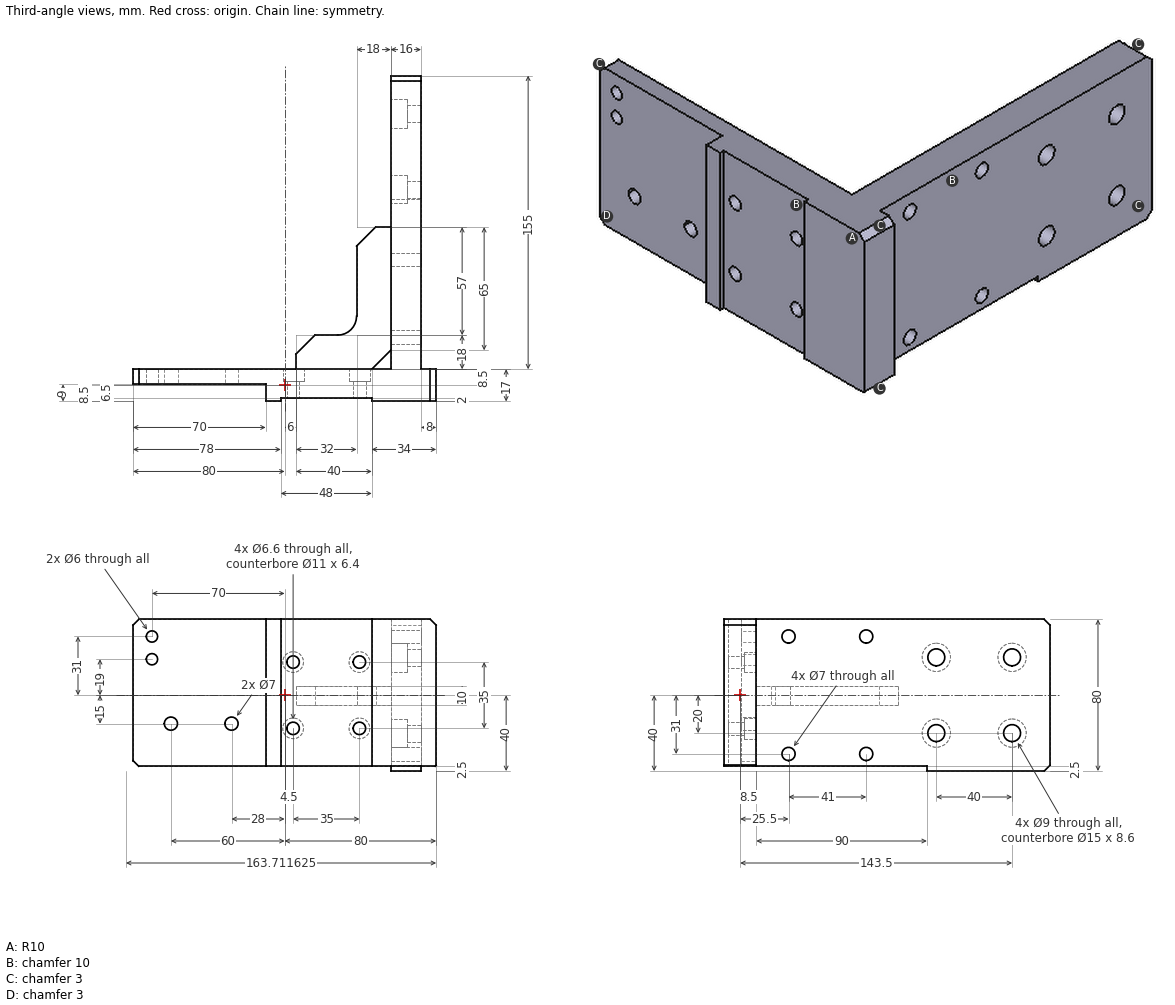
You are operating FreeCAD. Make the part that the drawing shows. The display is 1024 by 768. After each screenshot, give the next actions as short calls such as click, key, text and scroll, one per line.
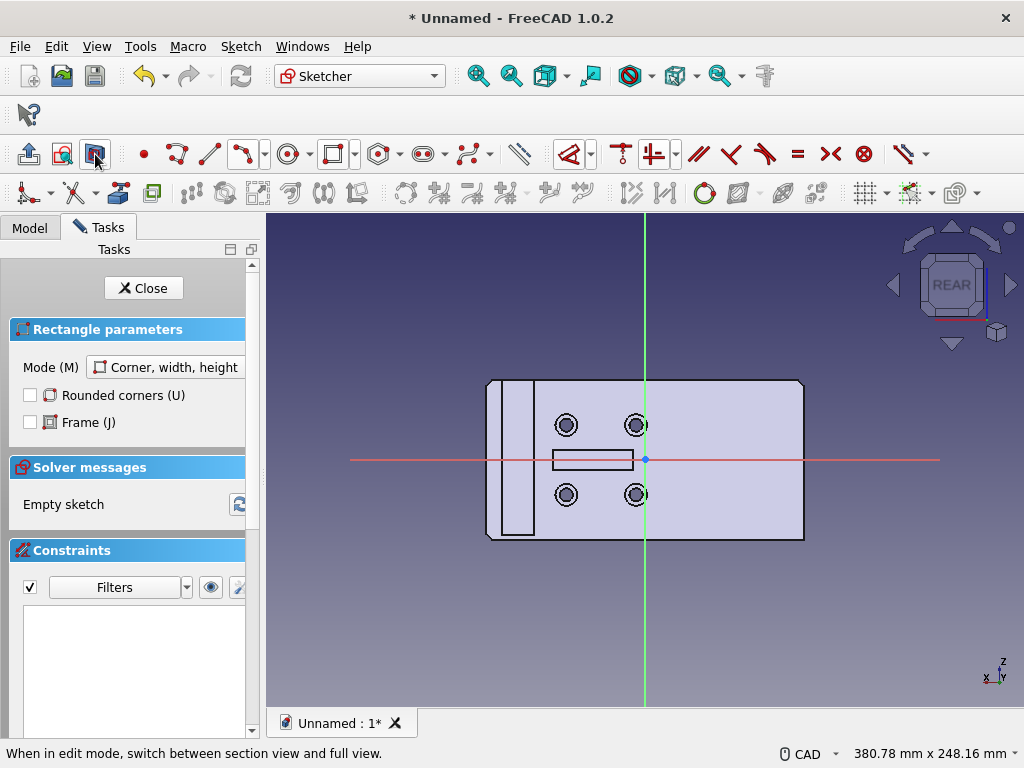
scroll(486, 535, up, 6)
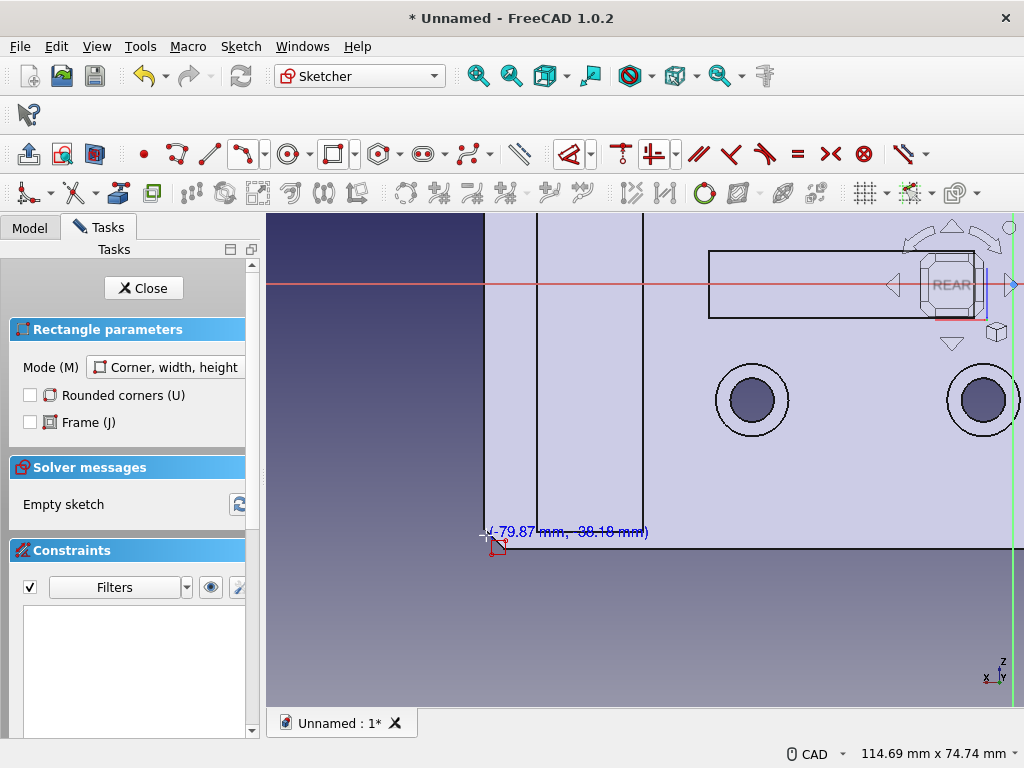
click(484, 532)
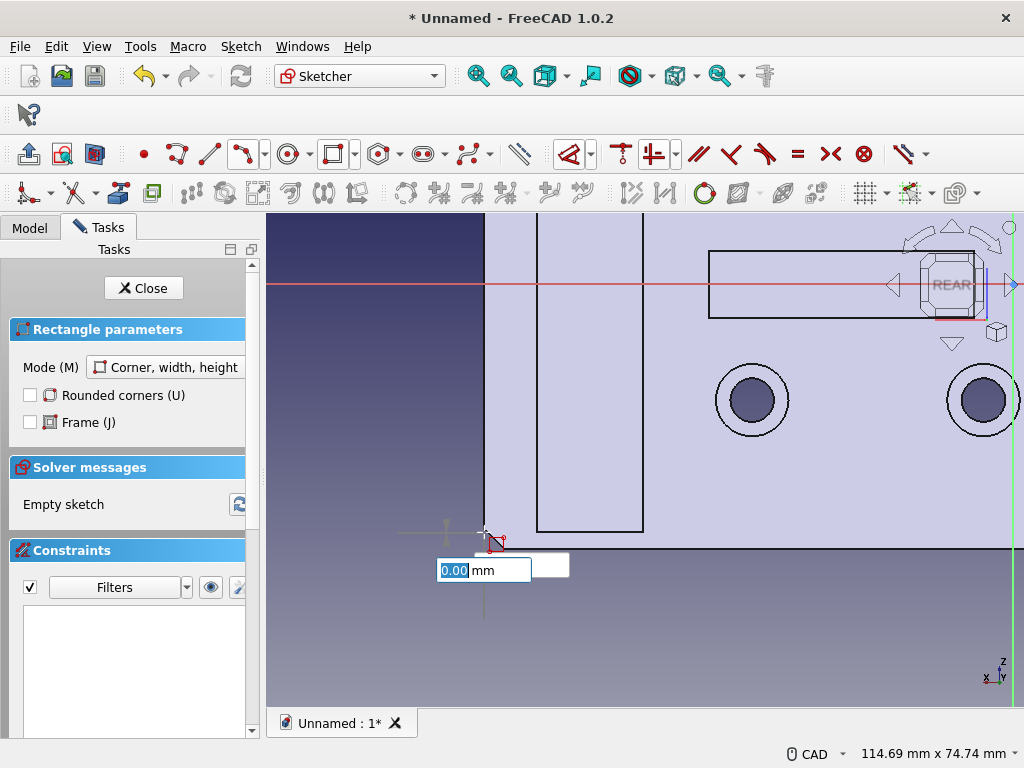
scroll(315, 485, down, 5)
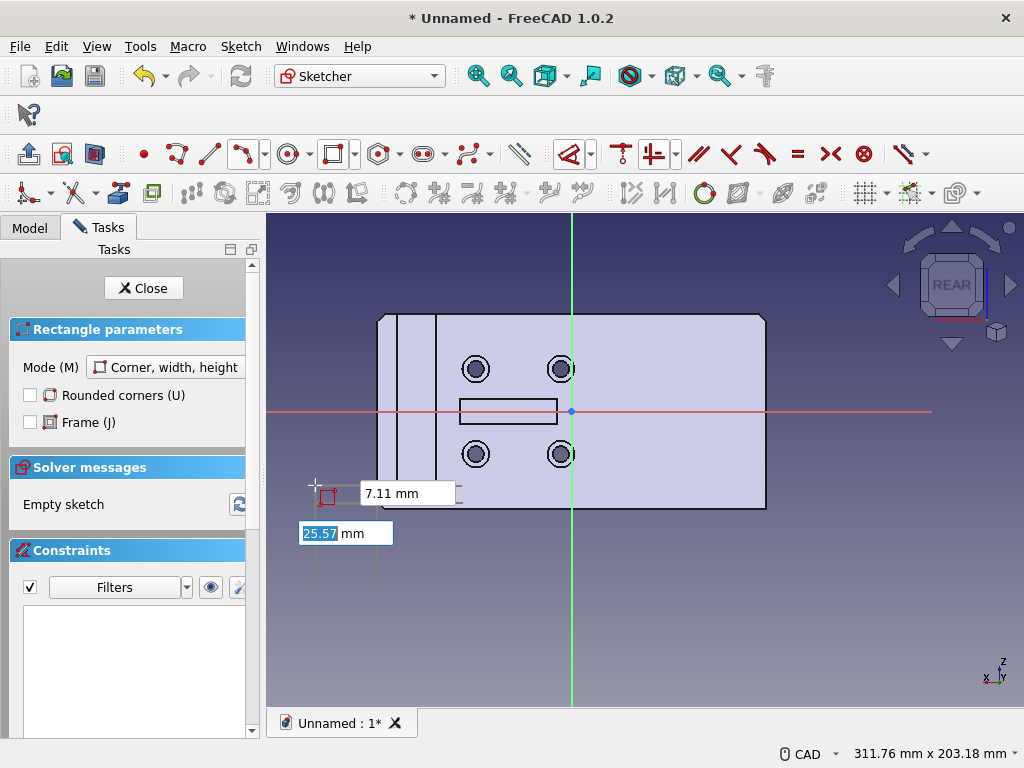
click(775, 509)
key(Escape)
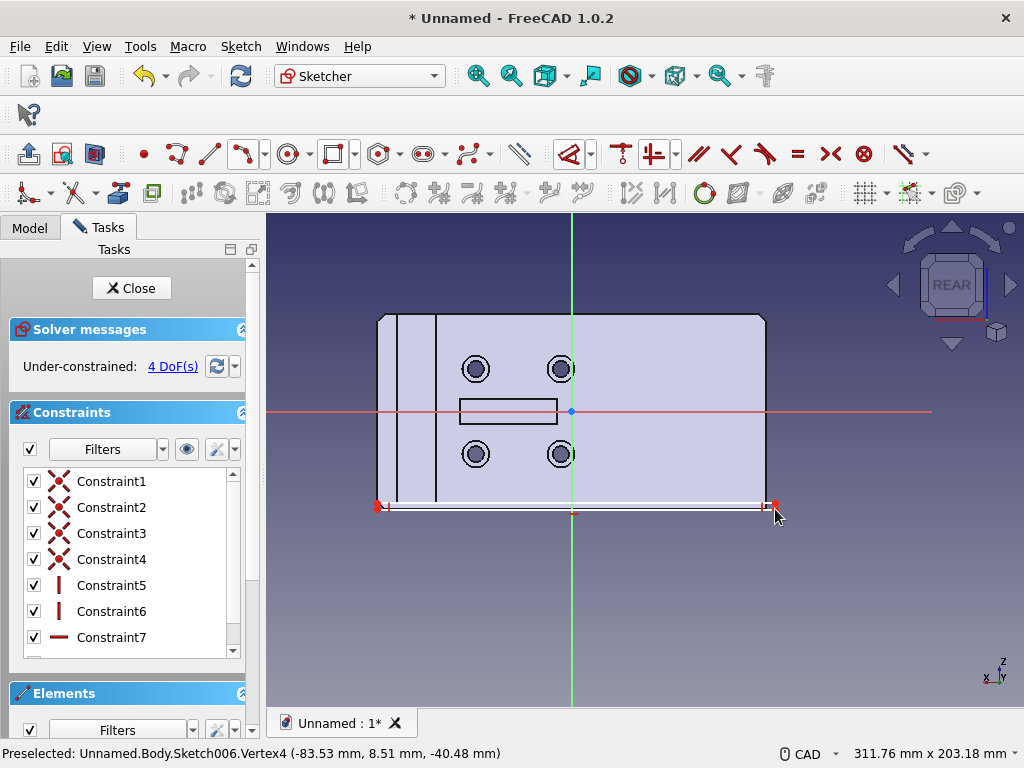
scroll(377, 507, up, 10)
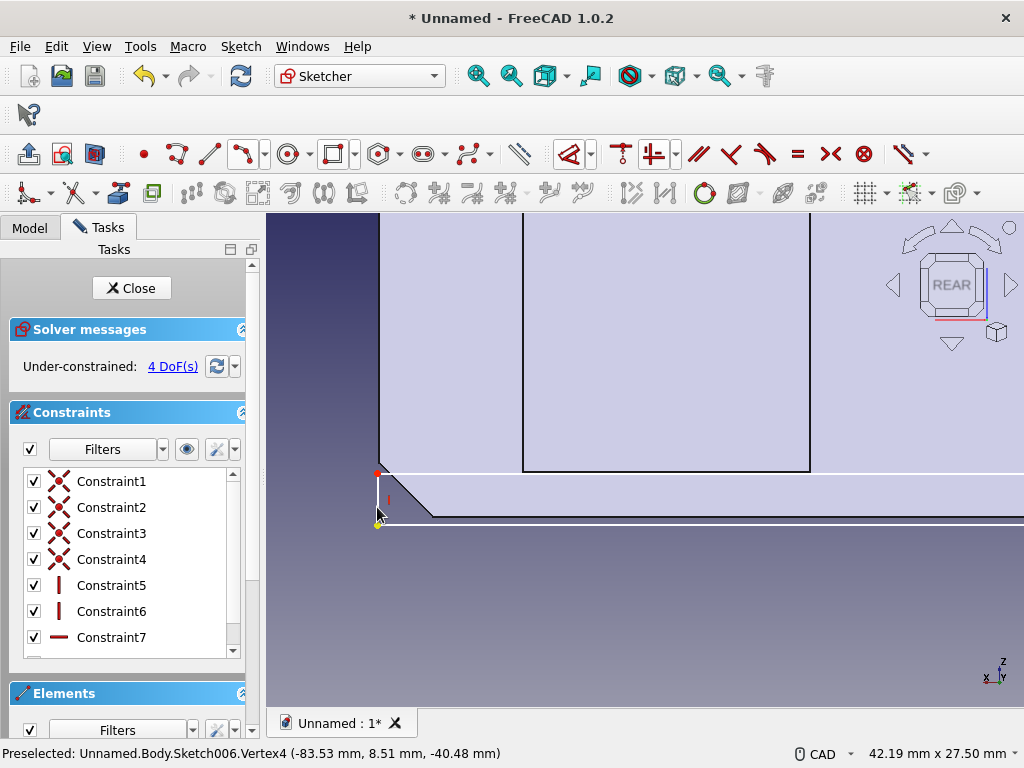
click(378, 500)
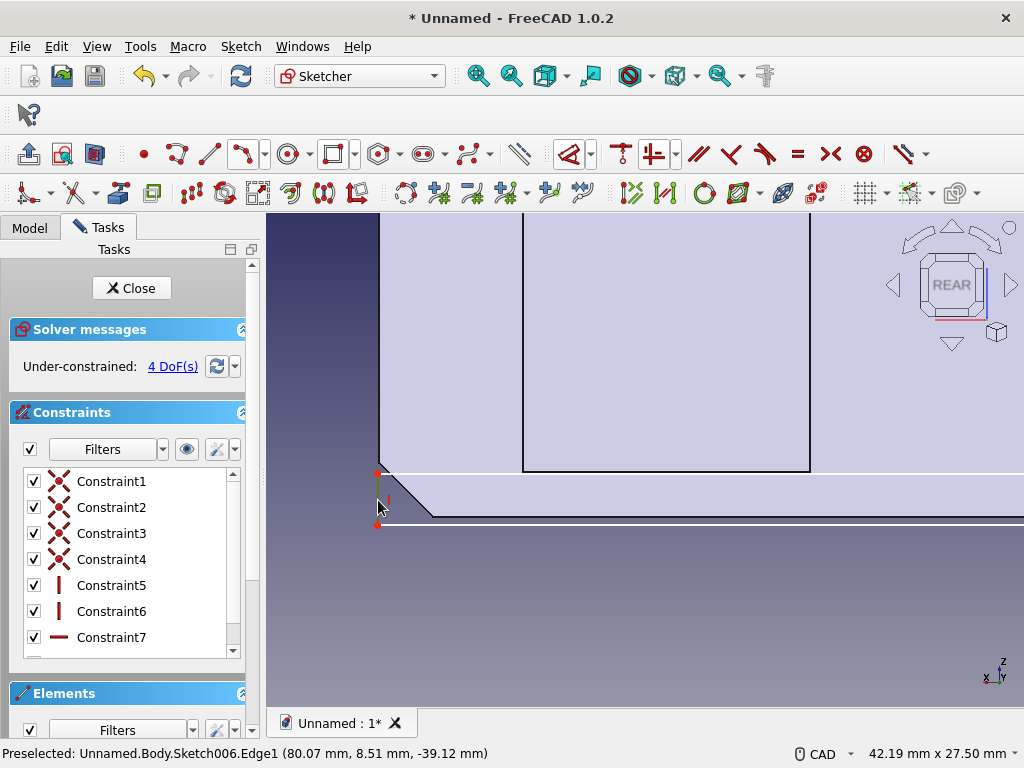
key(i)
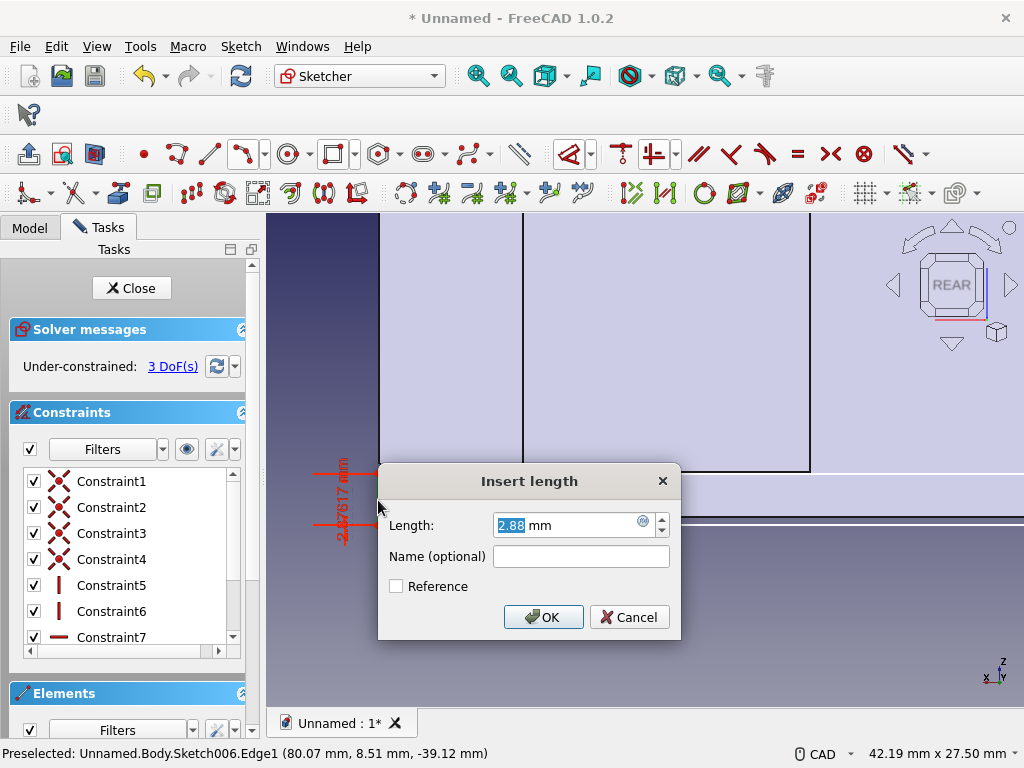
text(2.5)
key(Return)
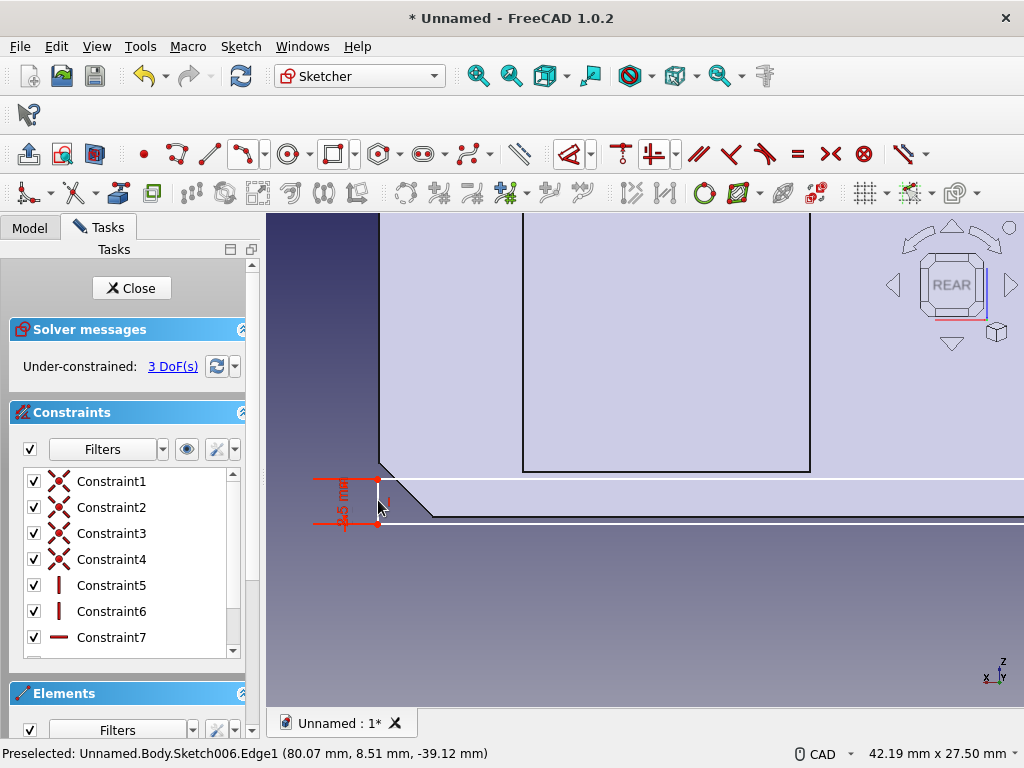
scroll(377, 507, down, 10)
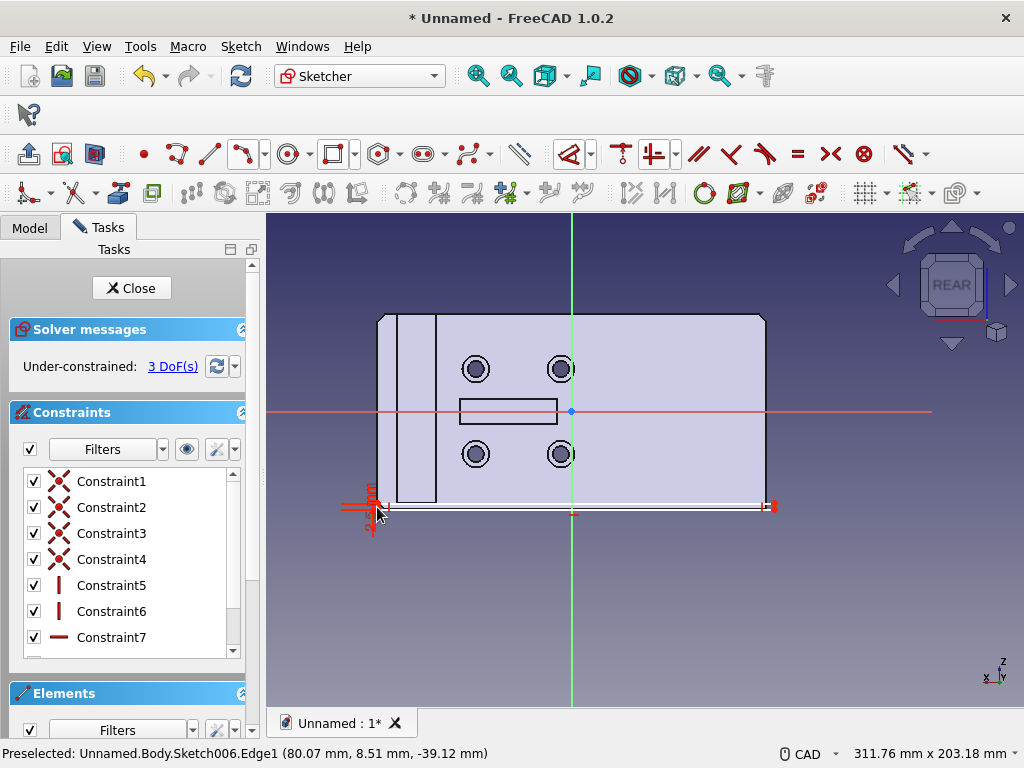
scroll(377, 504, up, 4)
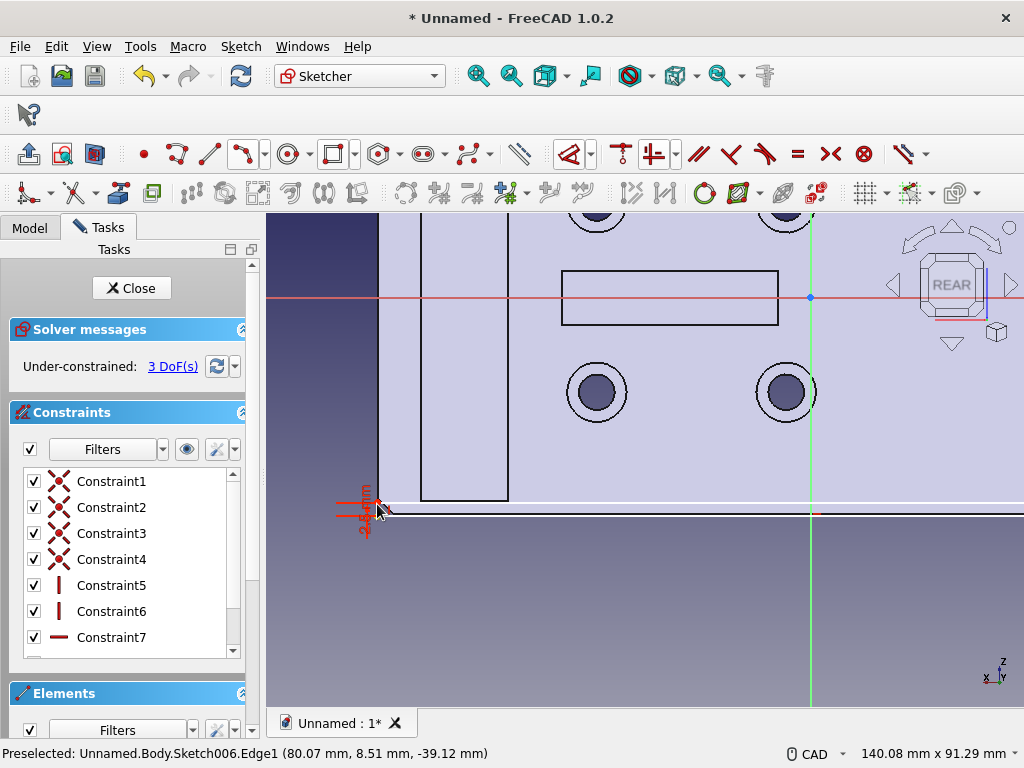
click(377, 503)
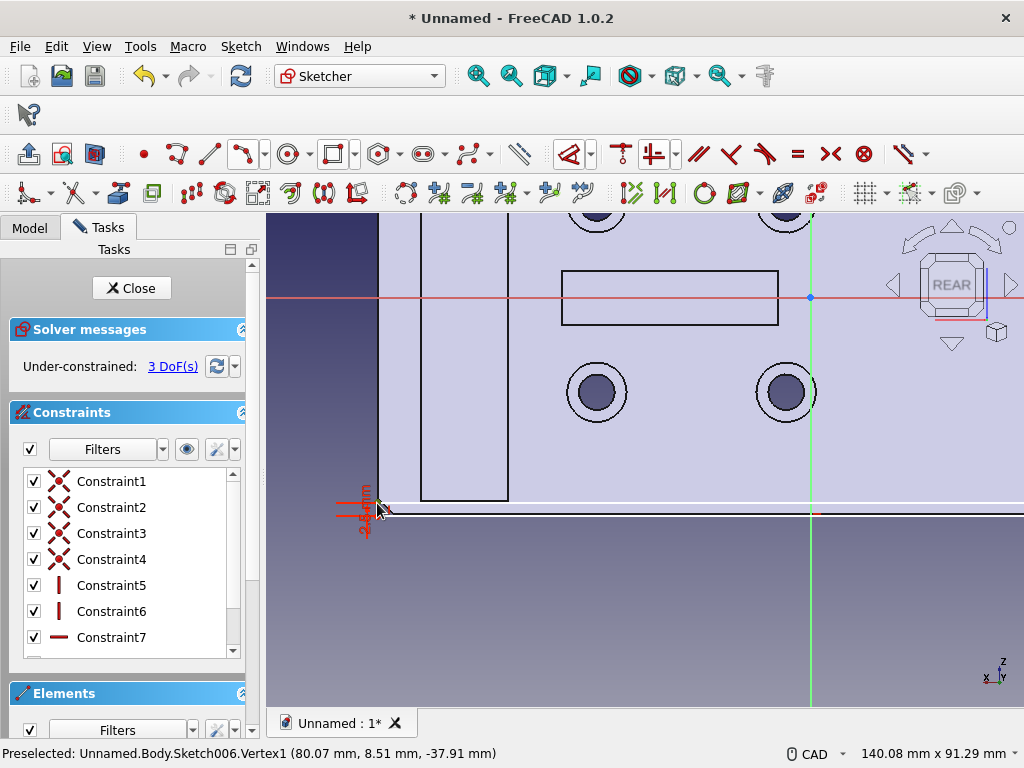
key(l)